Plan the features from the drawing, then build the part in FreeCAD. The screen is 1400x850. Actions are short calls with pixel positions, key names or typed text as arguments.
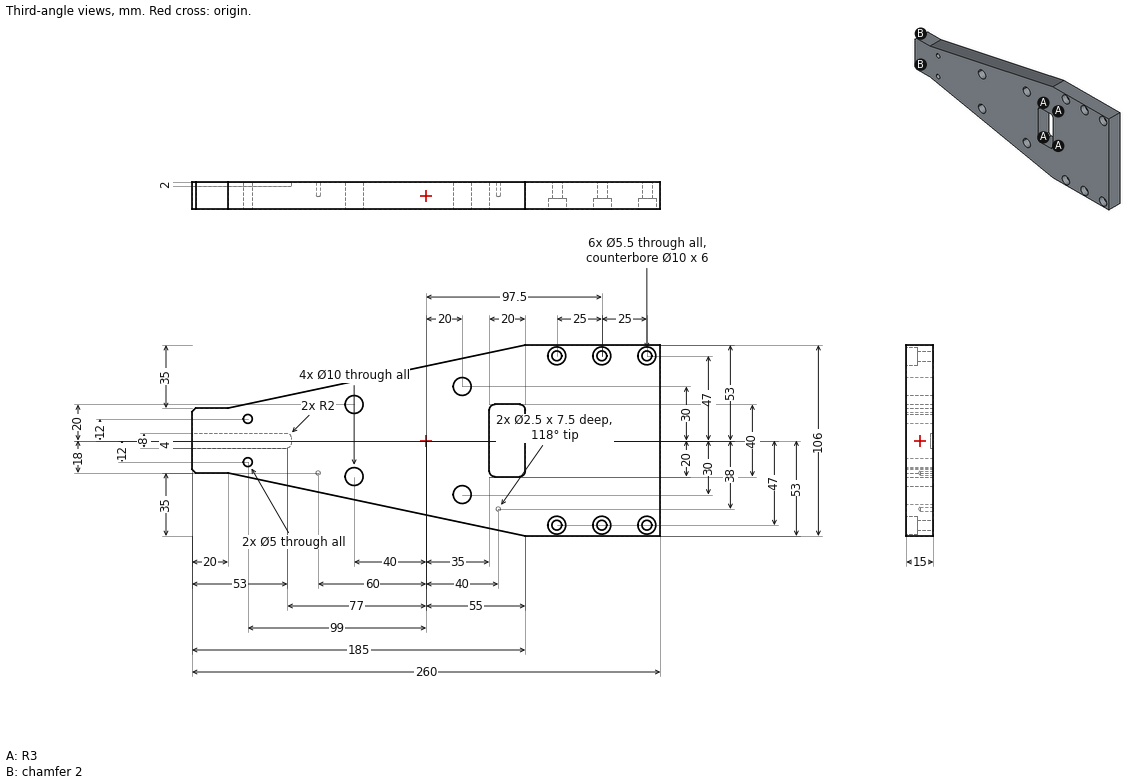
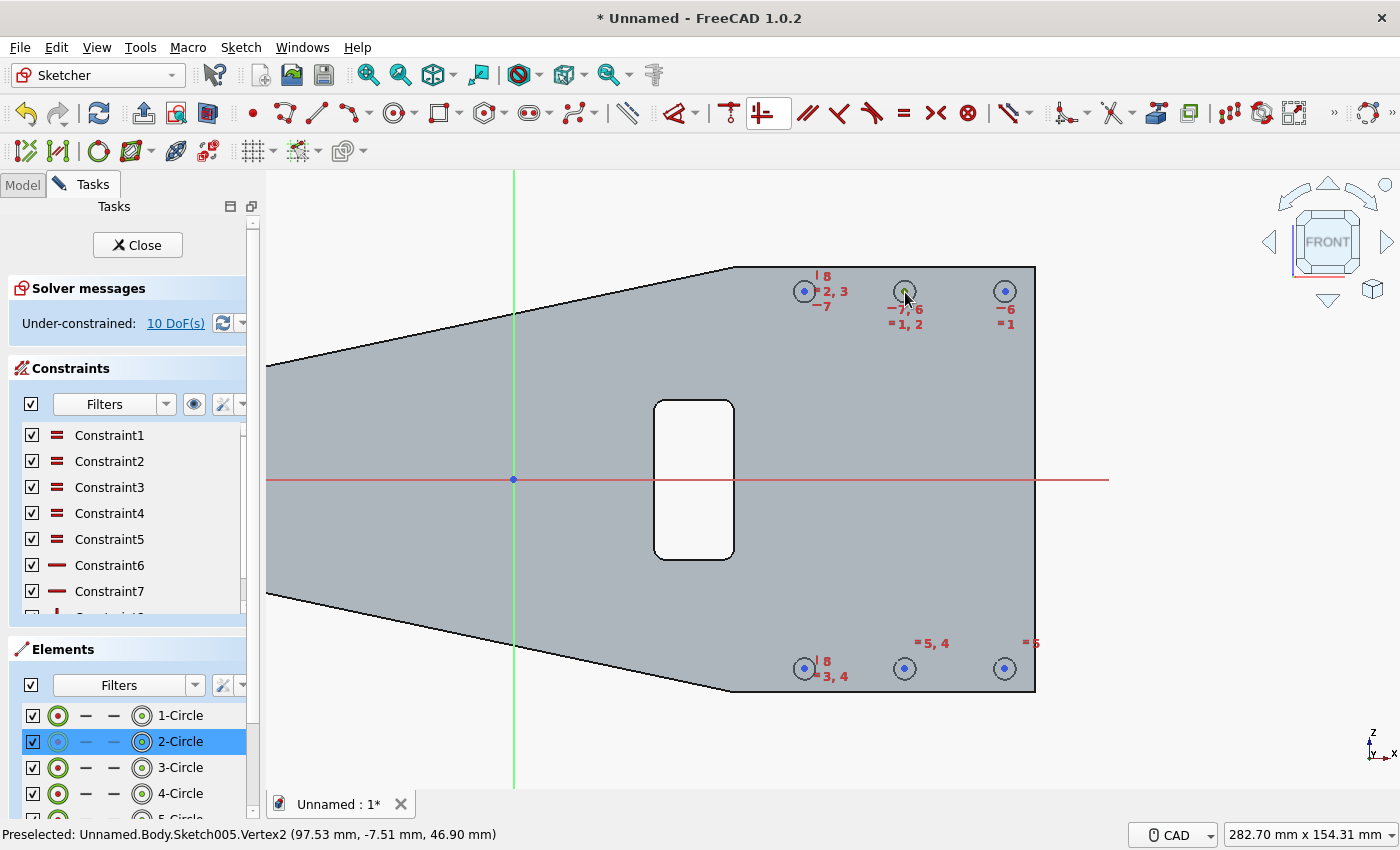
click(905, 669)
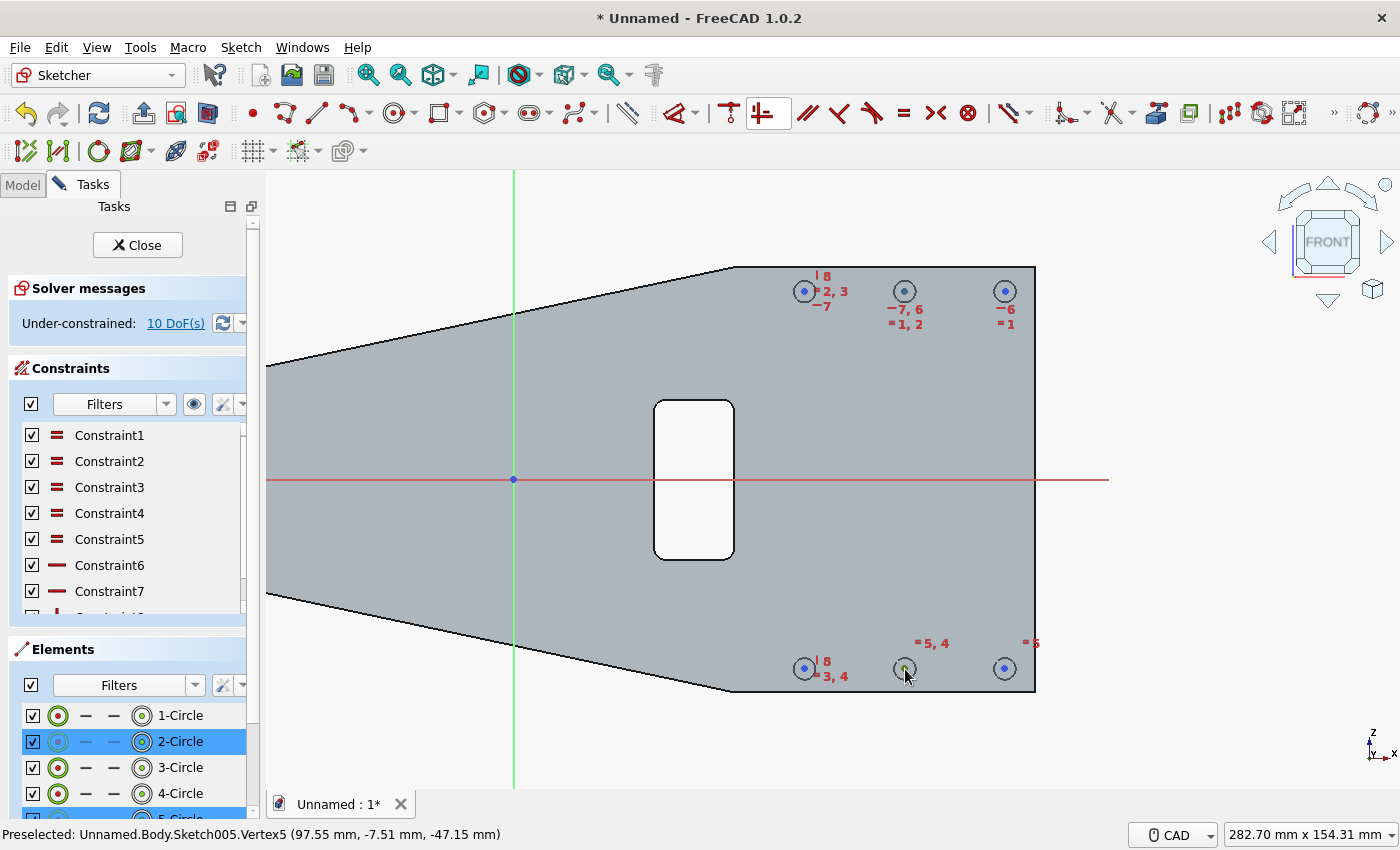
click(786, 114)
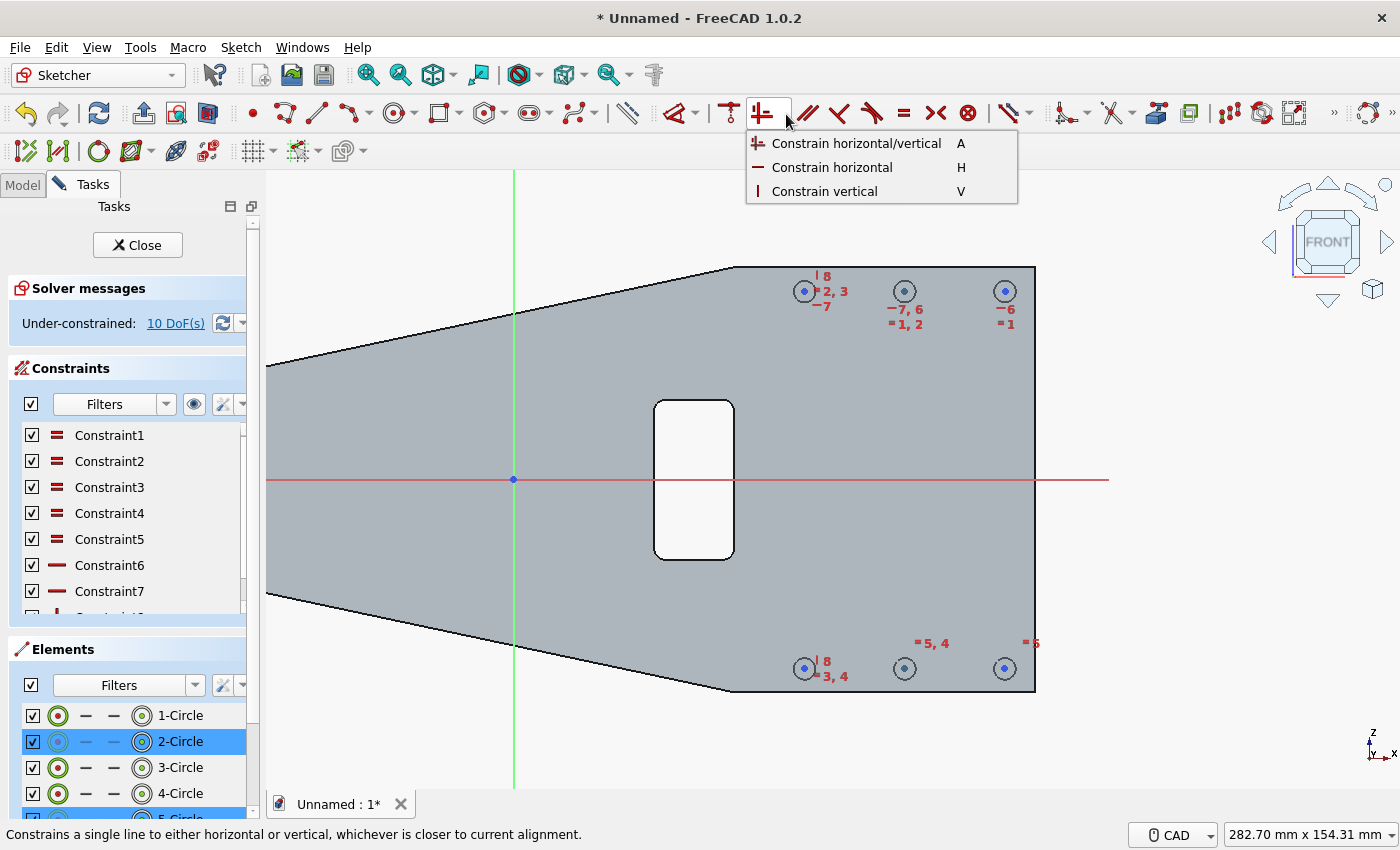
click(882, 191)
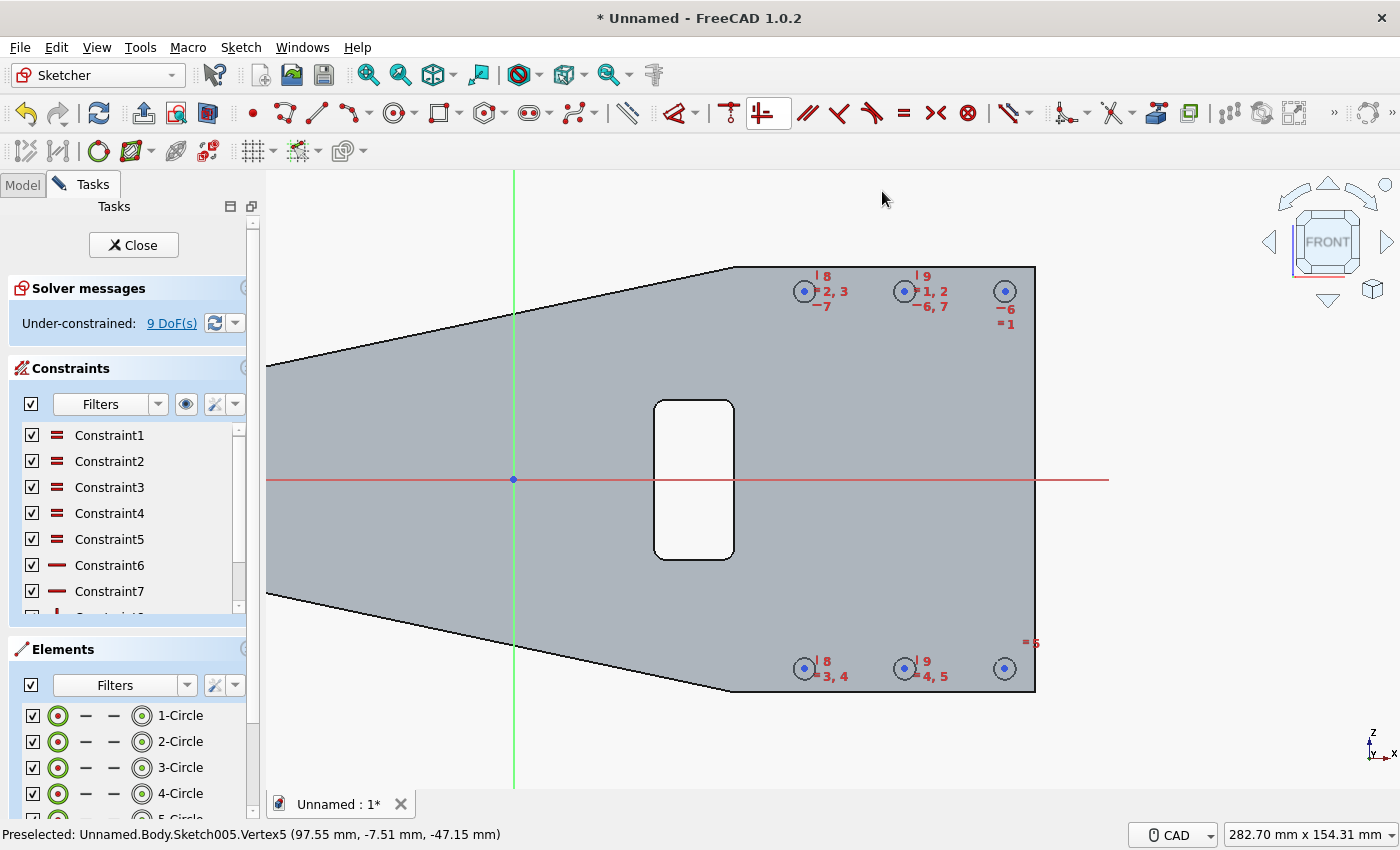
click(805, 669)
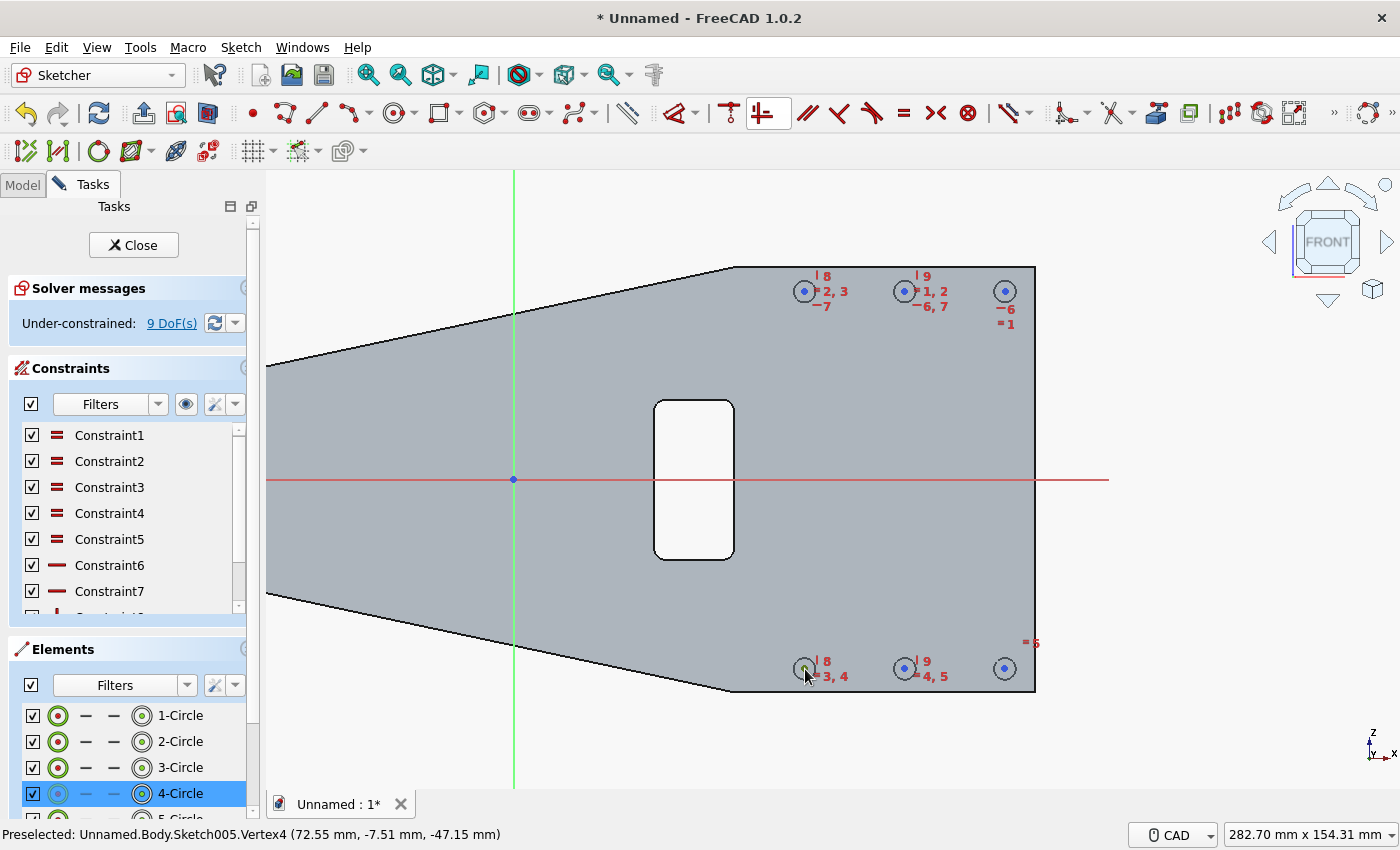
click(905, 669)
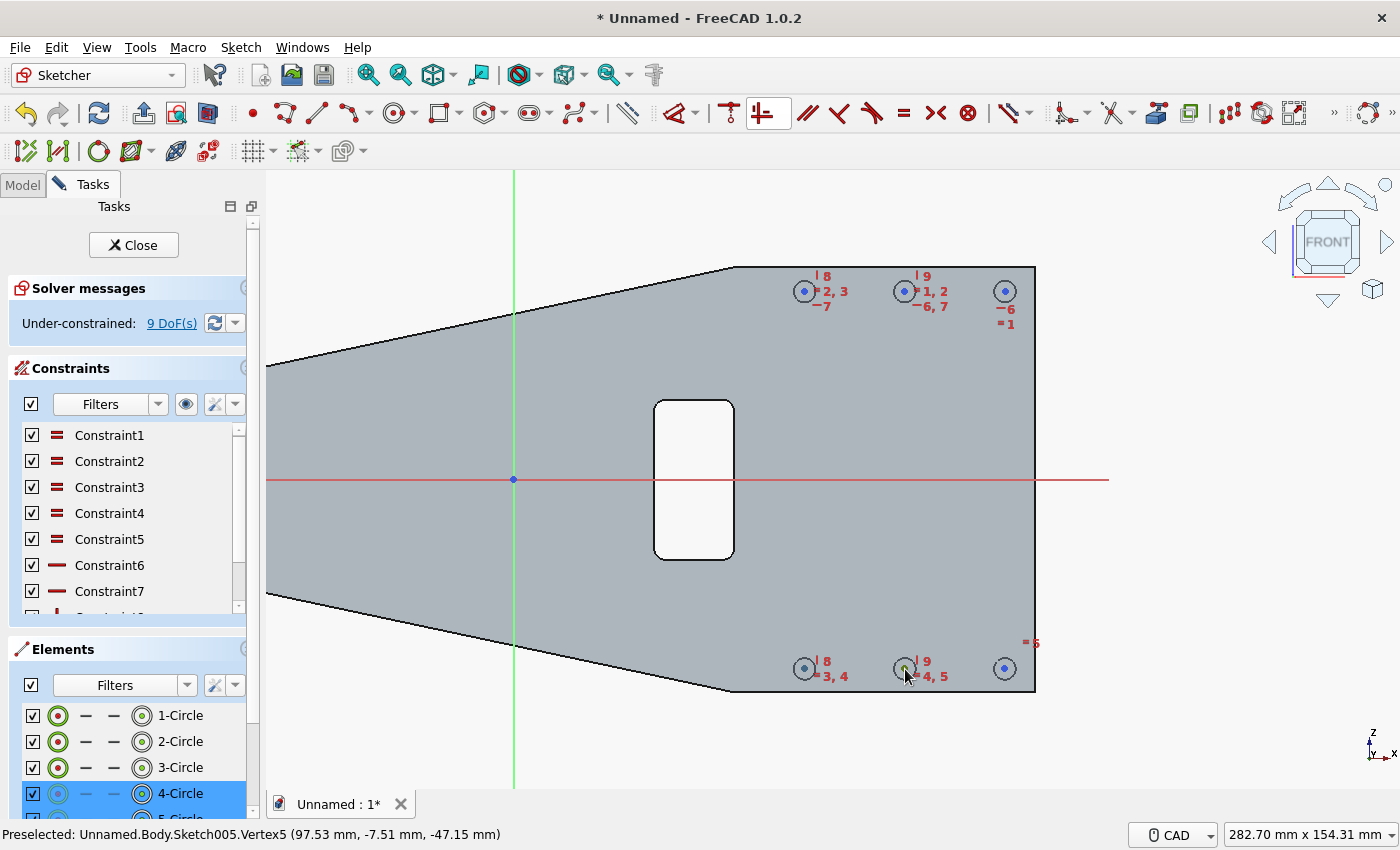
key(h)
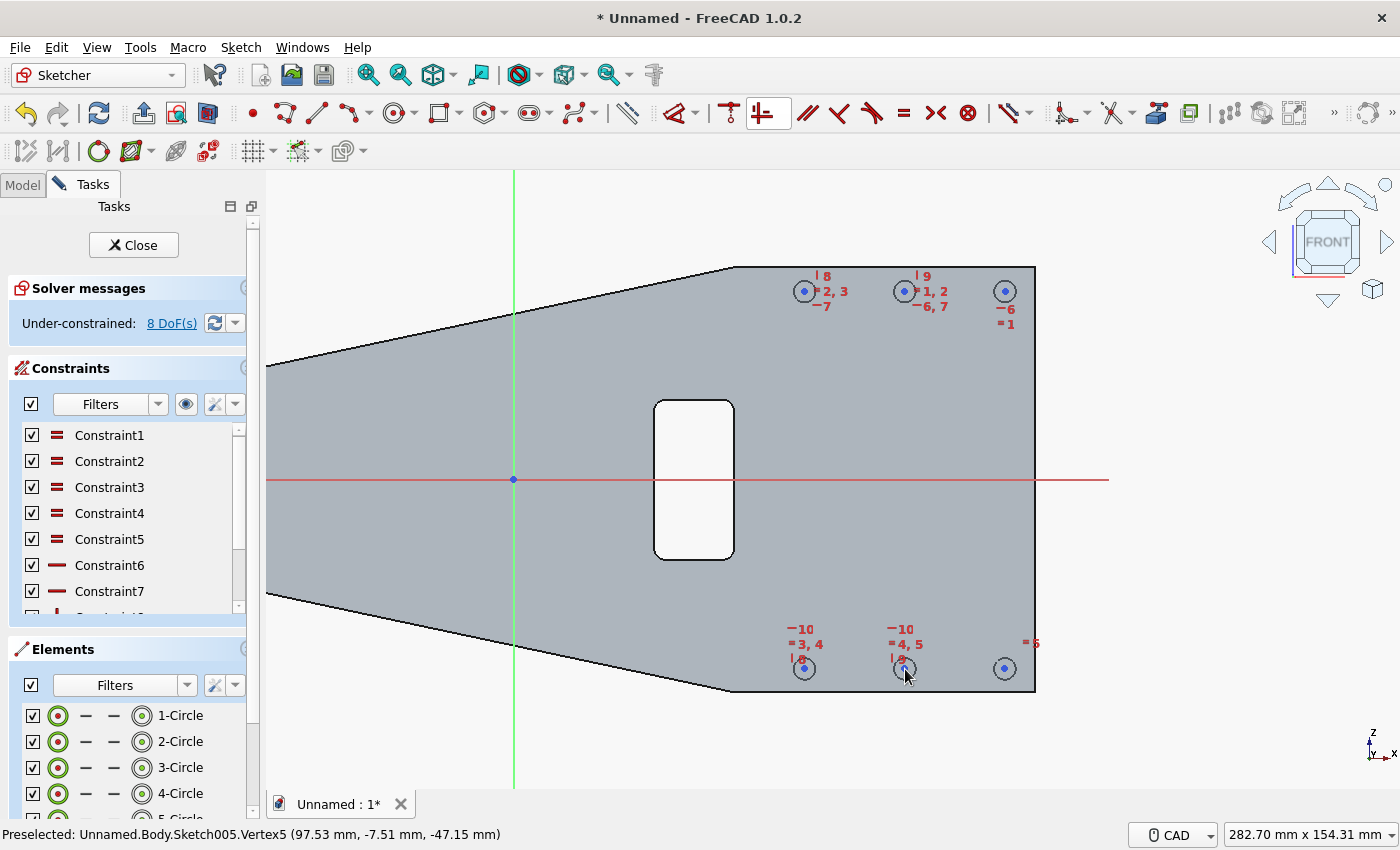
click(1005, 292)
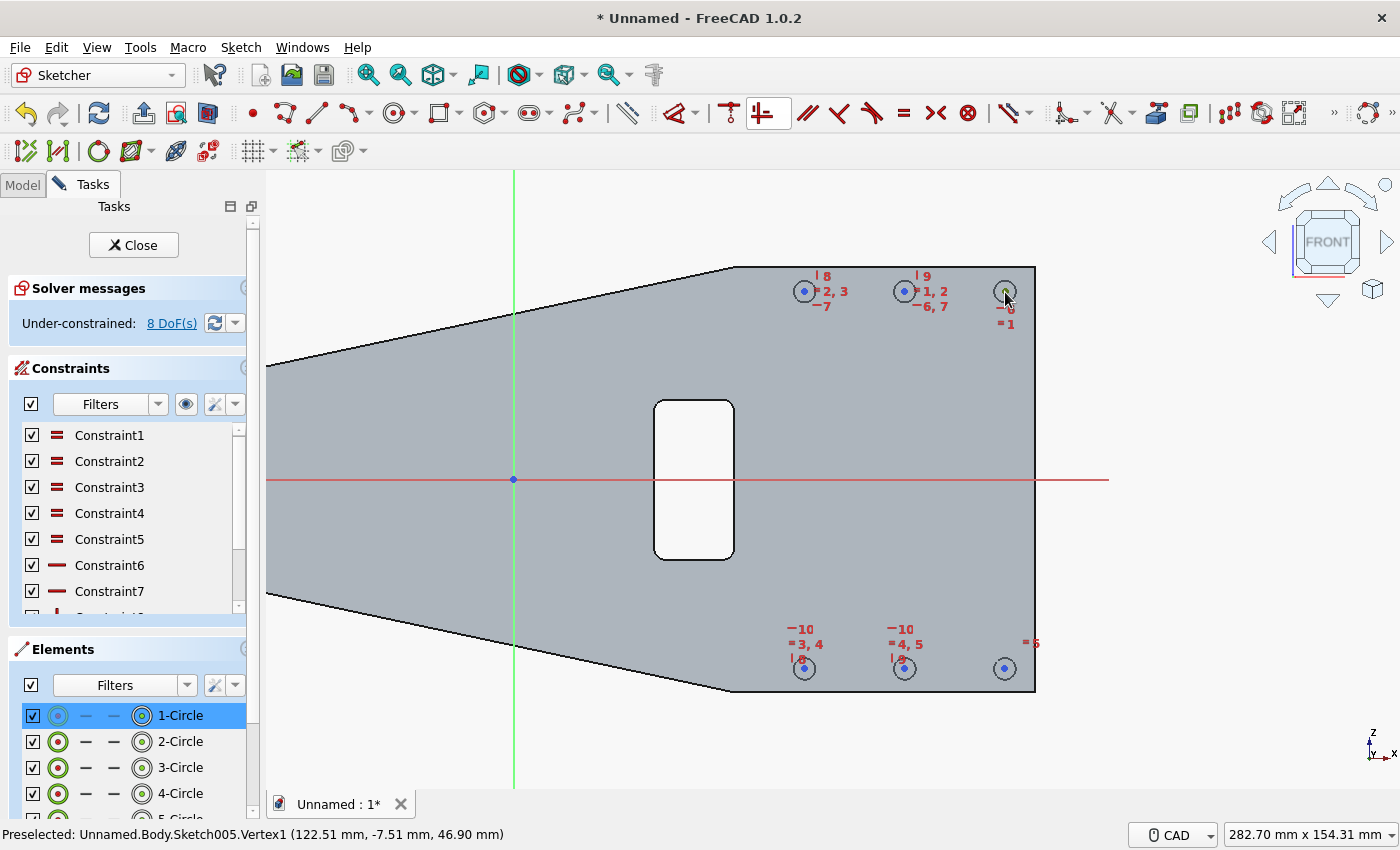
click(1005, 669)